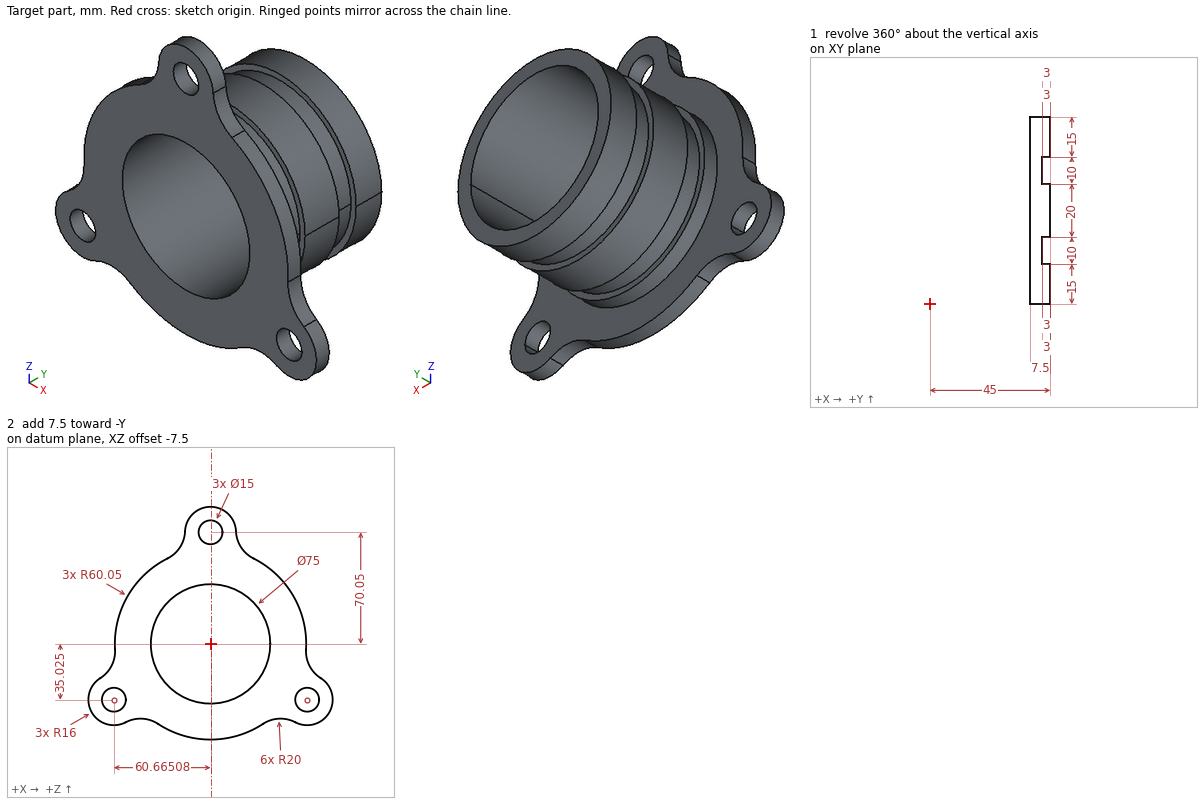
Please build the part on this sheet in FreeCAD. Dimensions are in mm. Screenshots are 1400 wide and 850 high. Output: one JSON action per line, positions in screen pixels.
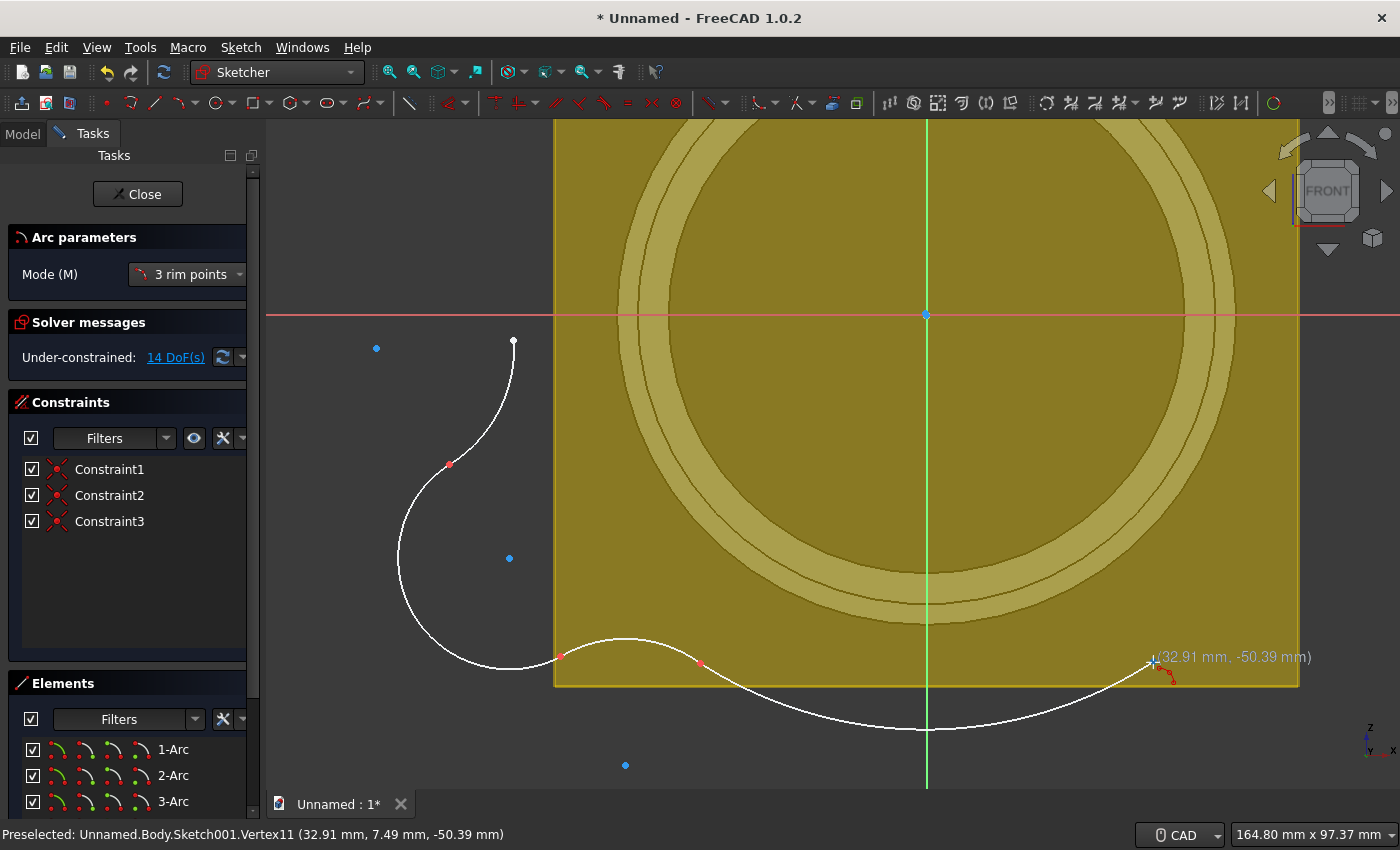
{"action": "scroll", "coordinate": [632, 640], "scroll_direction": "down", "scroll_amount": 4}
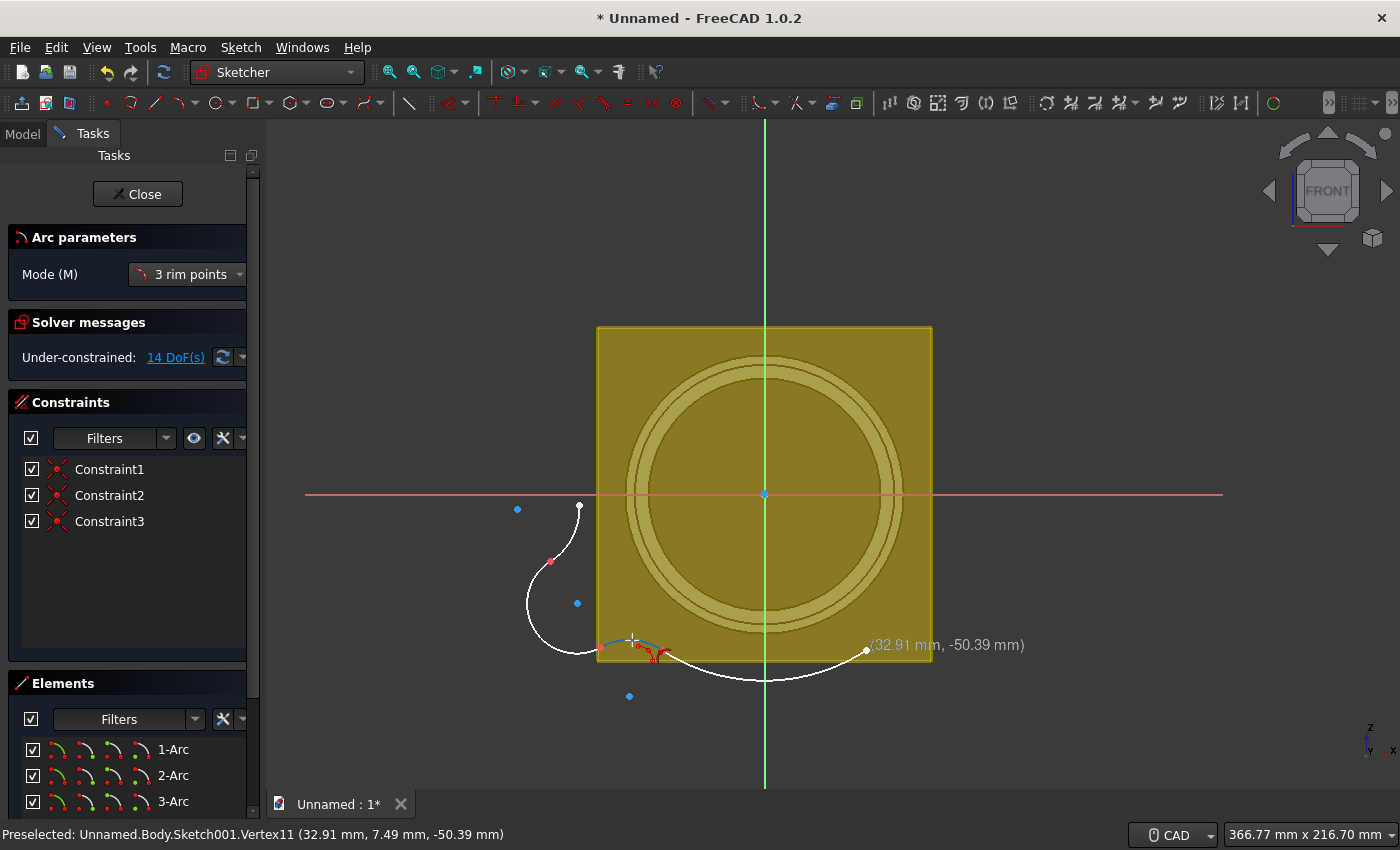
{"action": "left_click", "coordinate": [929, 647]}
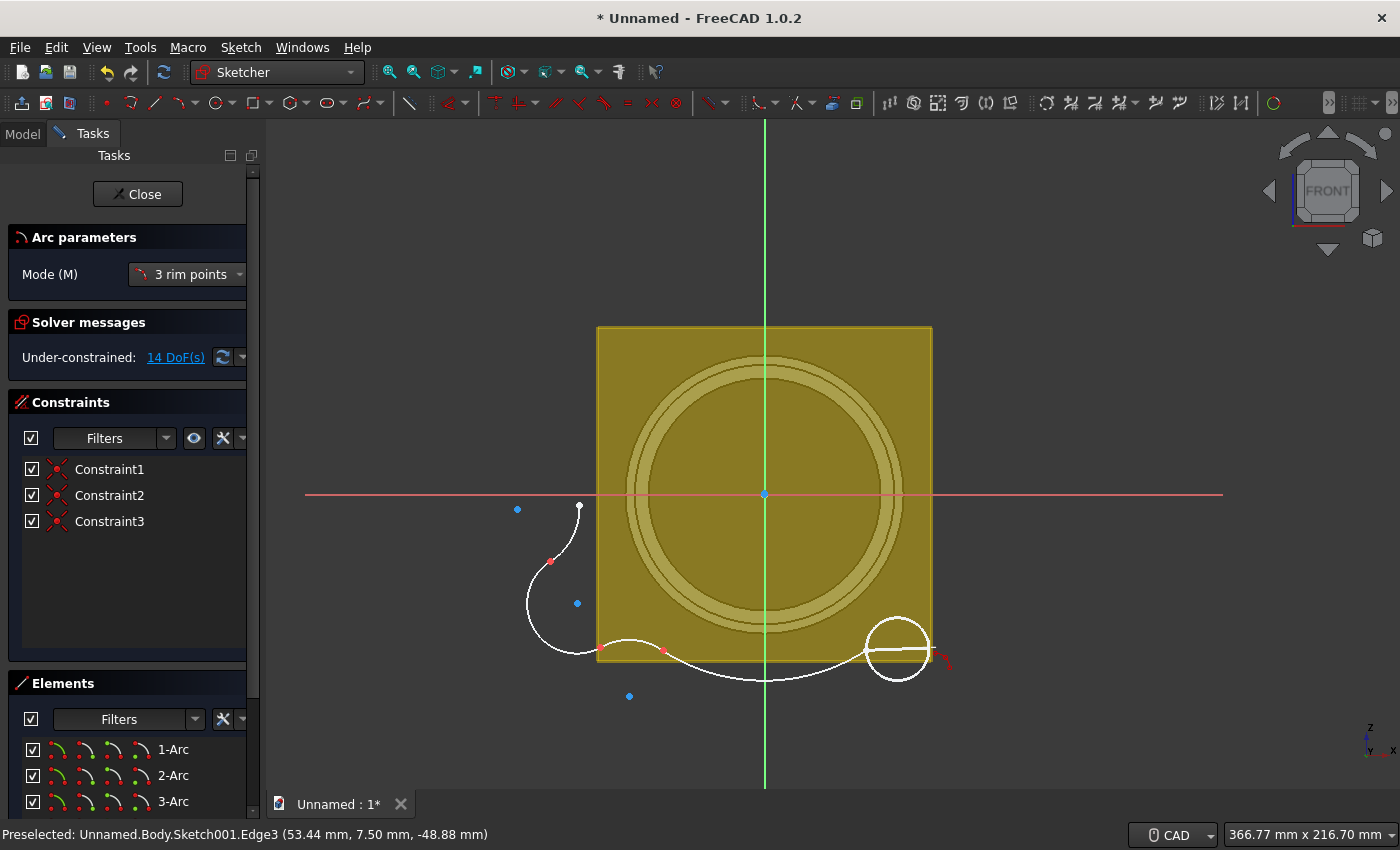
{"action": "scroll", "coordinate": [897, 640], "scroll_direction": "up", "scroll_amount": 4}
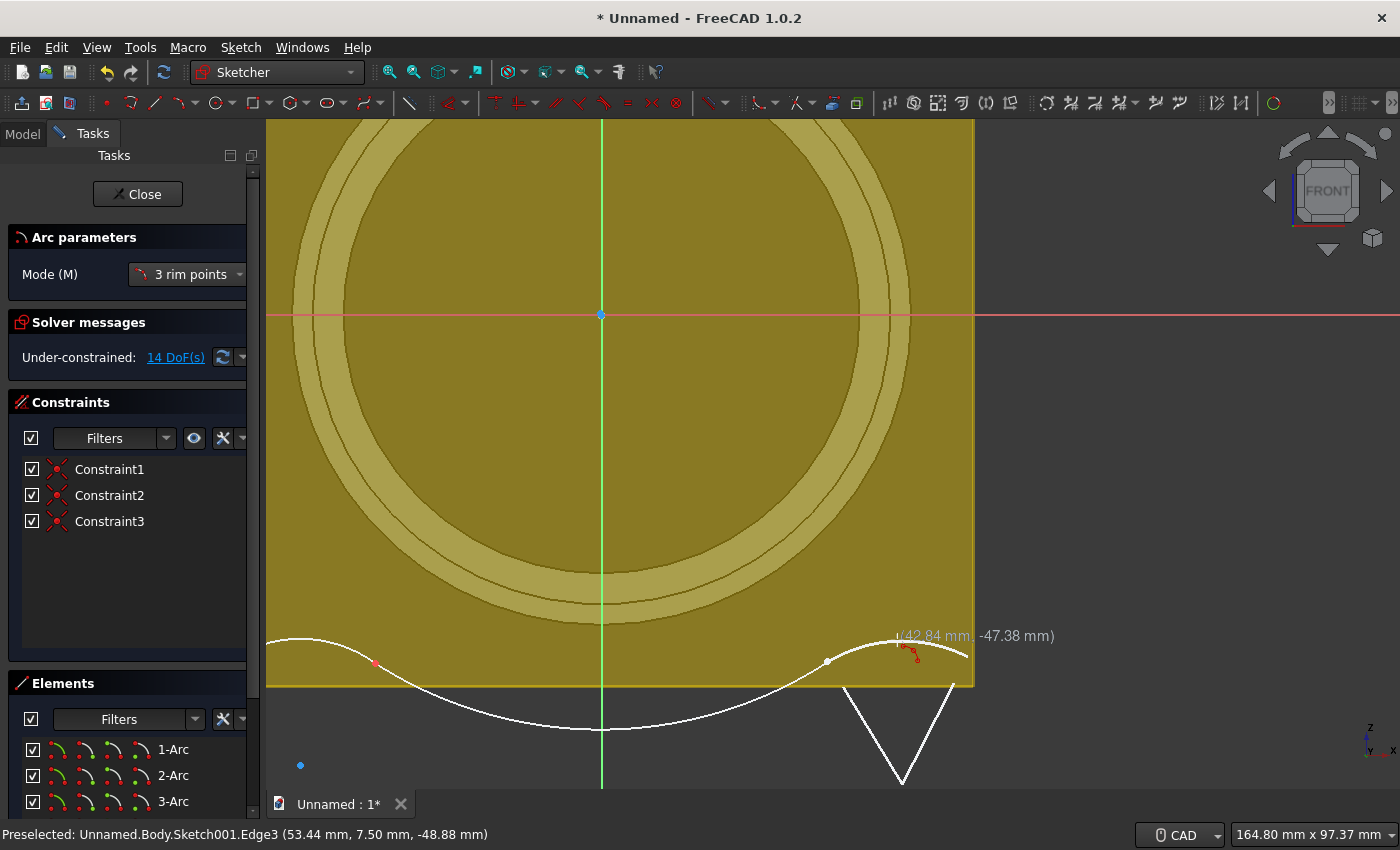
{"action": "left_click", "coordinate": [897, 638]}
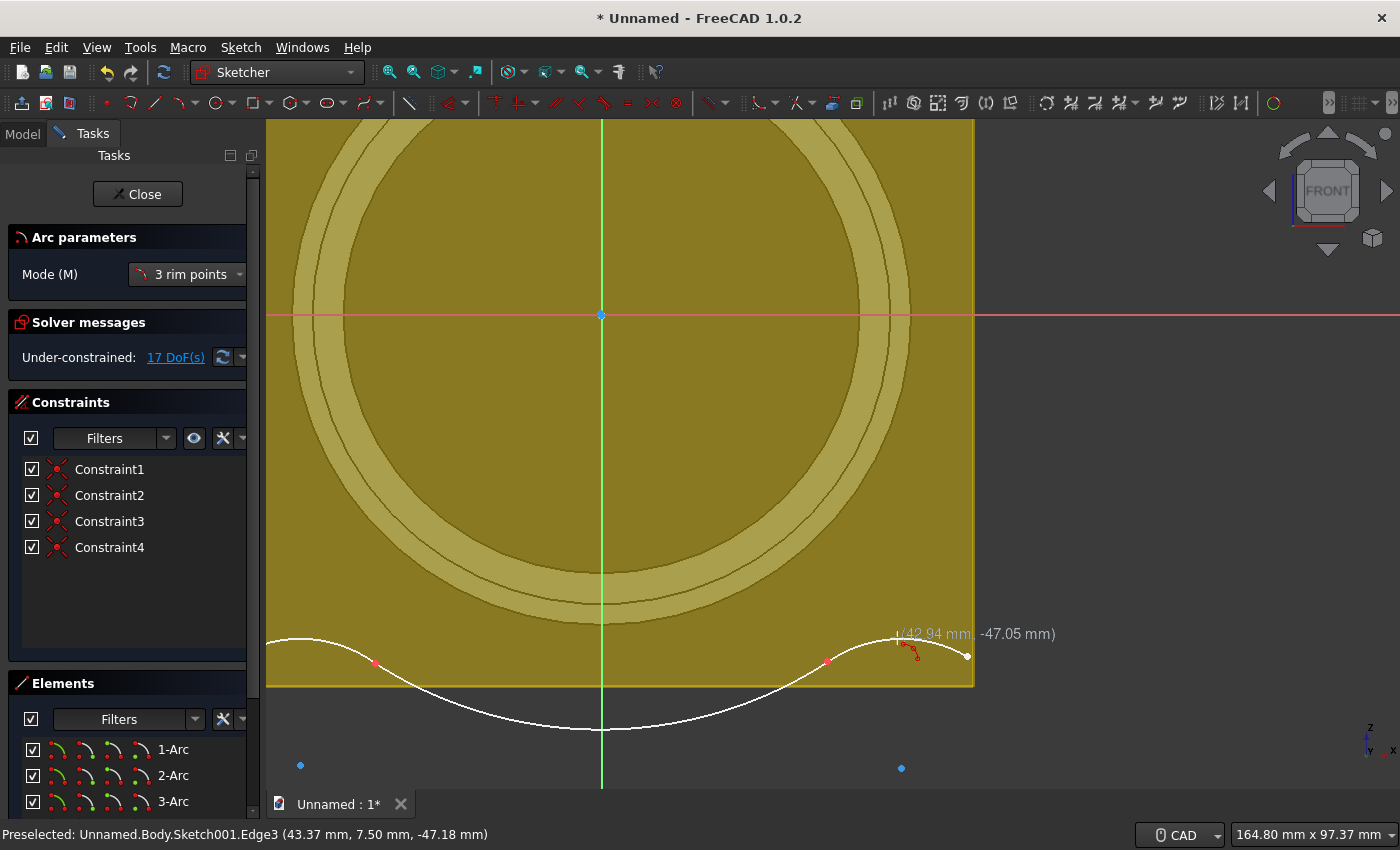
{"action": "left_click", "coordinate": [968, 657]}
{"action": "left_click", "coordinate": [1078, 463]}
{"action": "left_click", "coordinate": [1114, 611]}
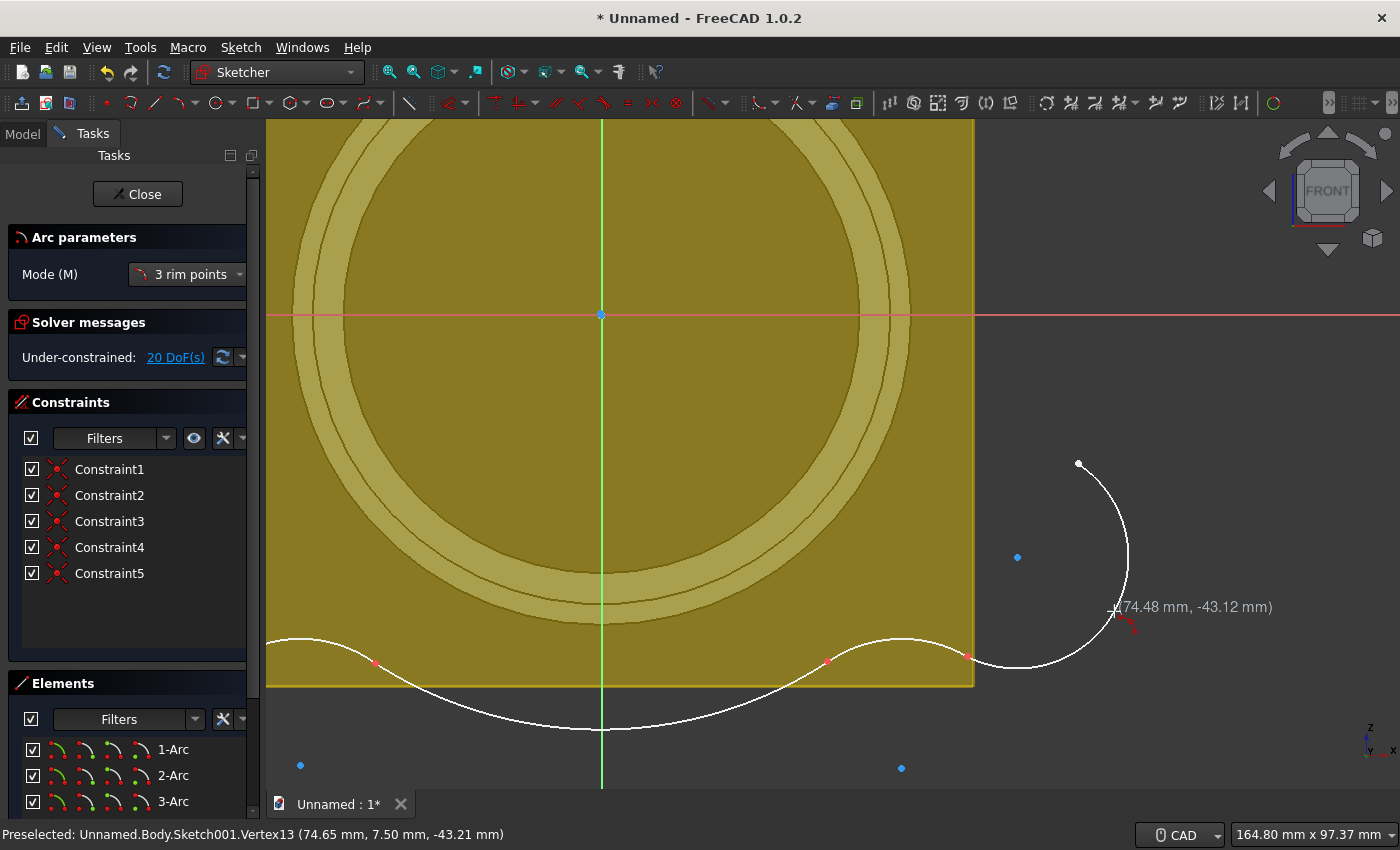
{"action": "left_click", "coordinate": [1078, 464]}
{"action": "left_click", "coordinate": [1014, 339]}
{"action": "left_click", "coordinate": [1029, 410]}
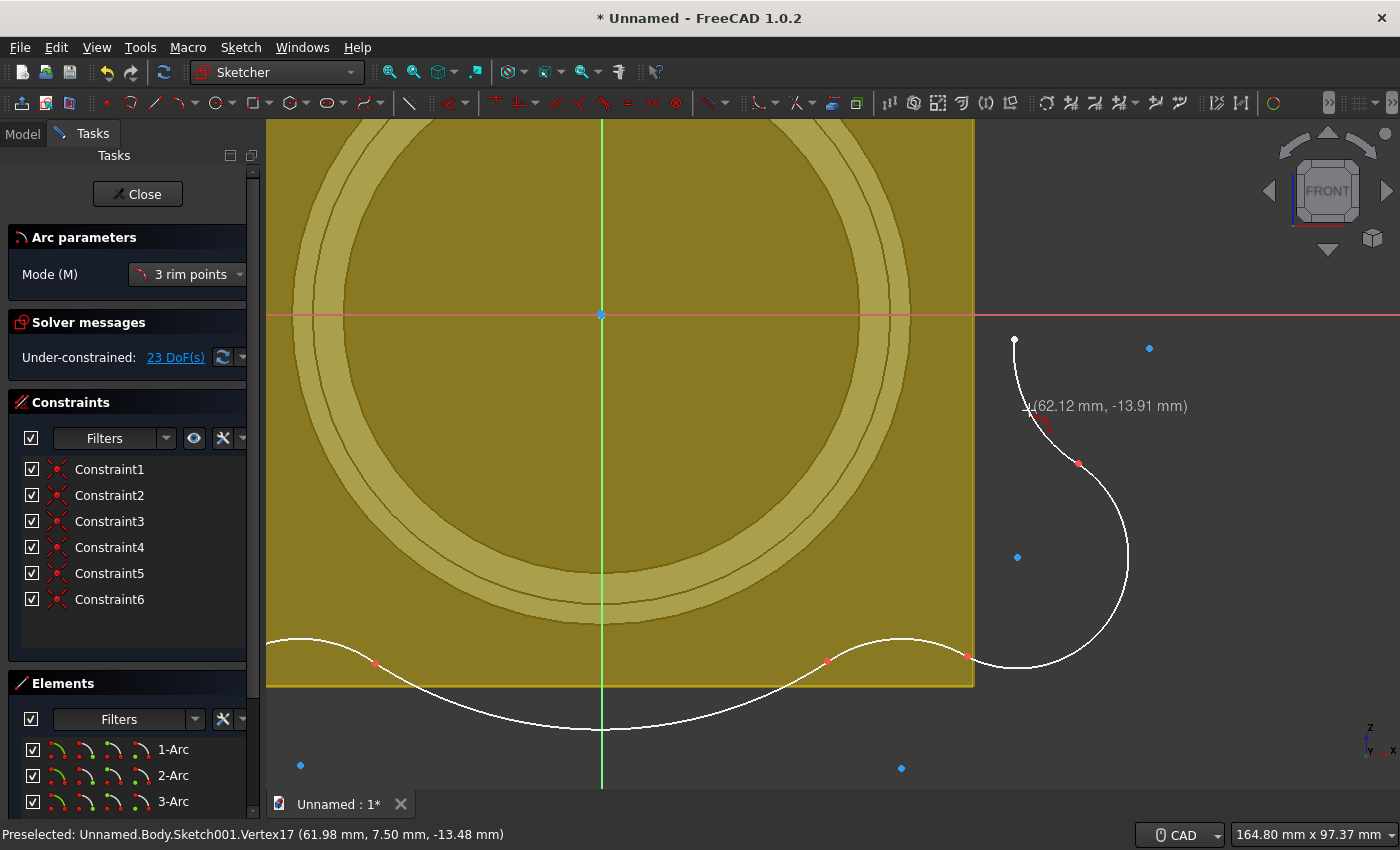
{"action": "left_click", "coordinate": [1014, 340]}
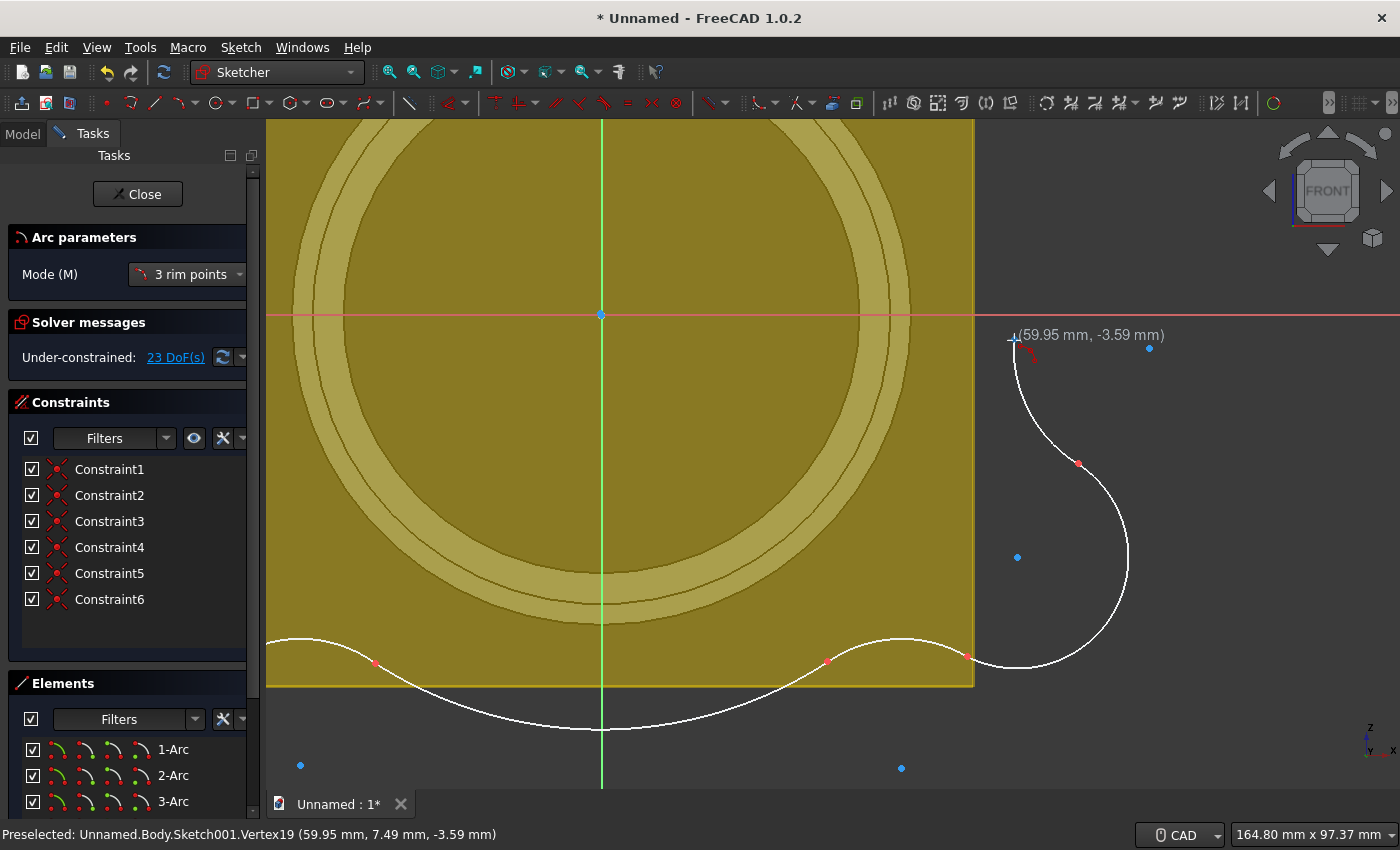
{"action": "scroll", "coordinate": [897, 640], "scroll_direction": "down", "scroll_amount": 4}